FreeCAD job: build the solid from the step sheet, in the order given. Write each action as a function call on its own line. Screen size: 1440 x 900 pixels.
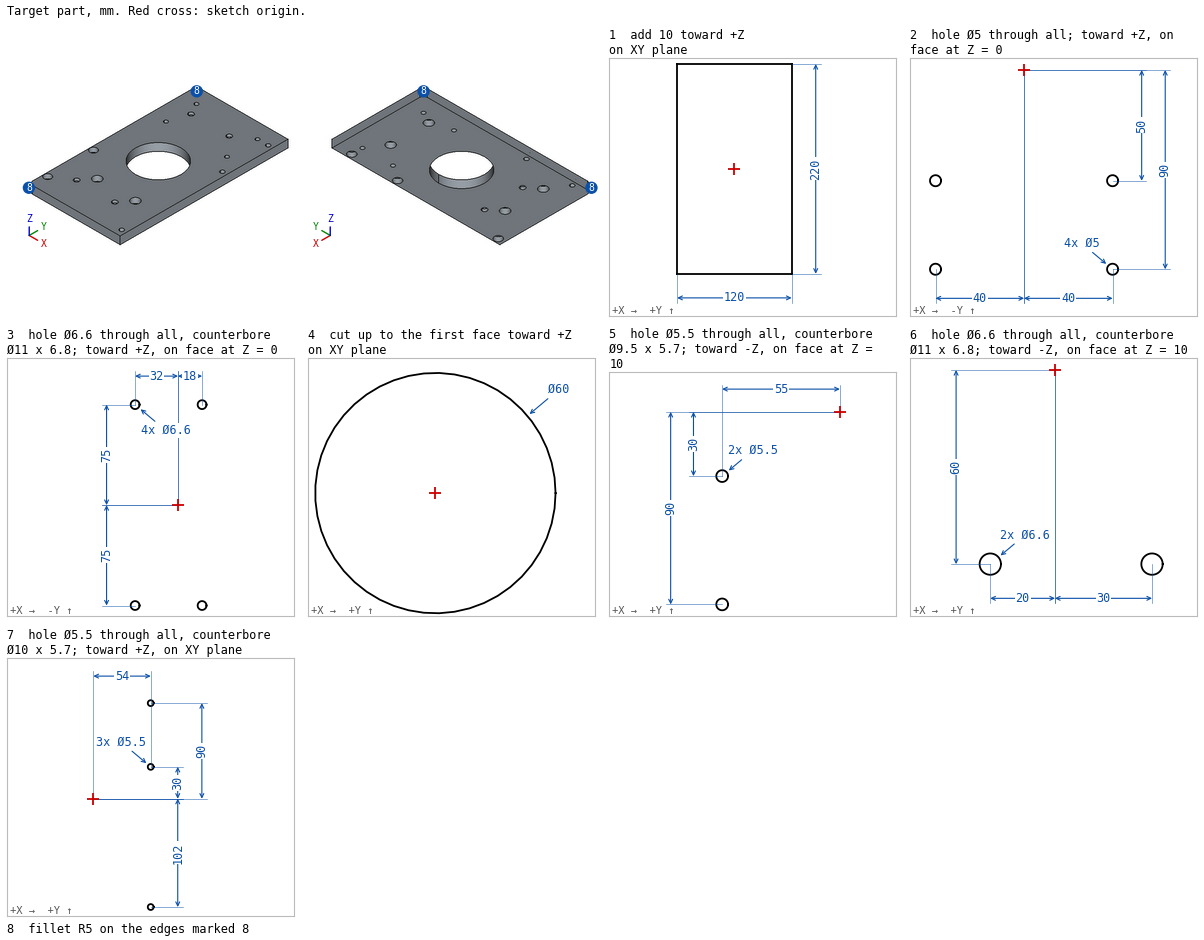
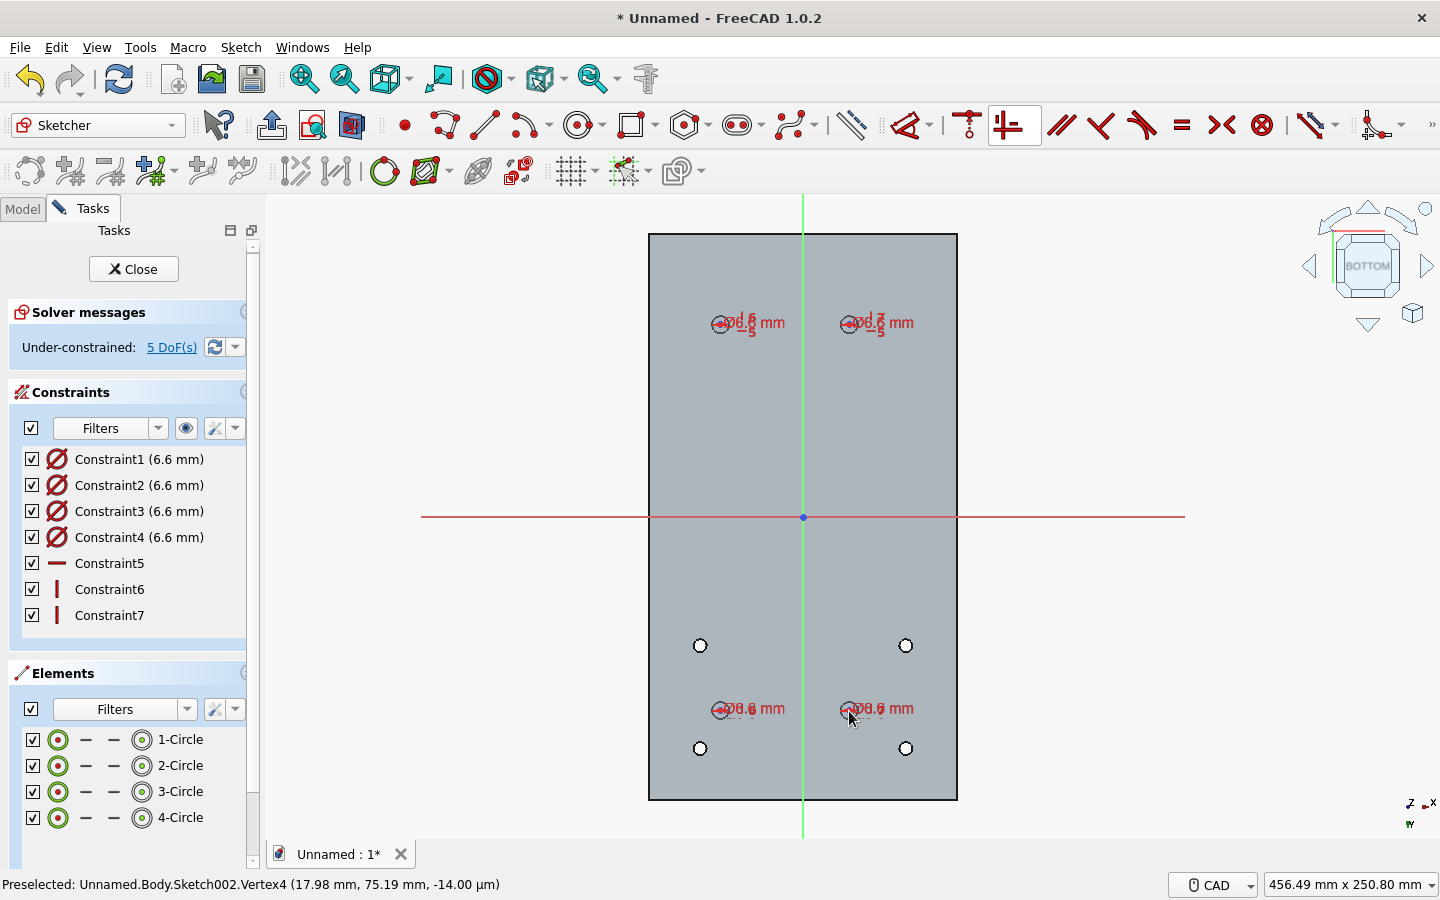
click(721, 711)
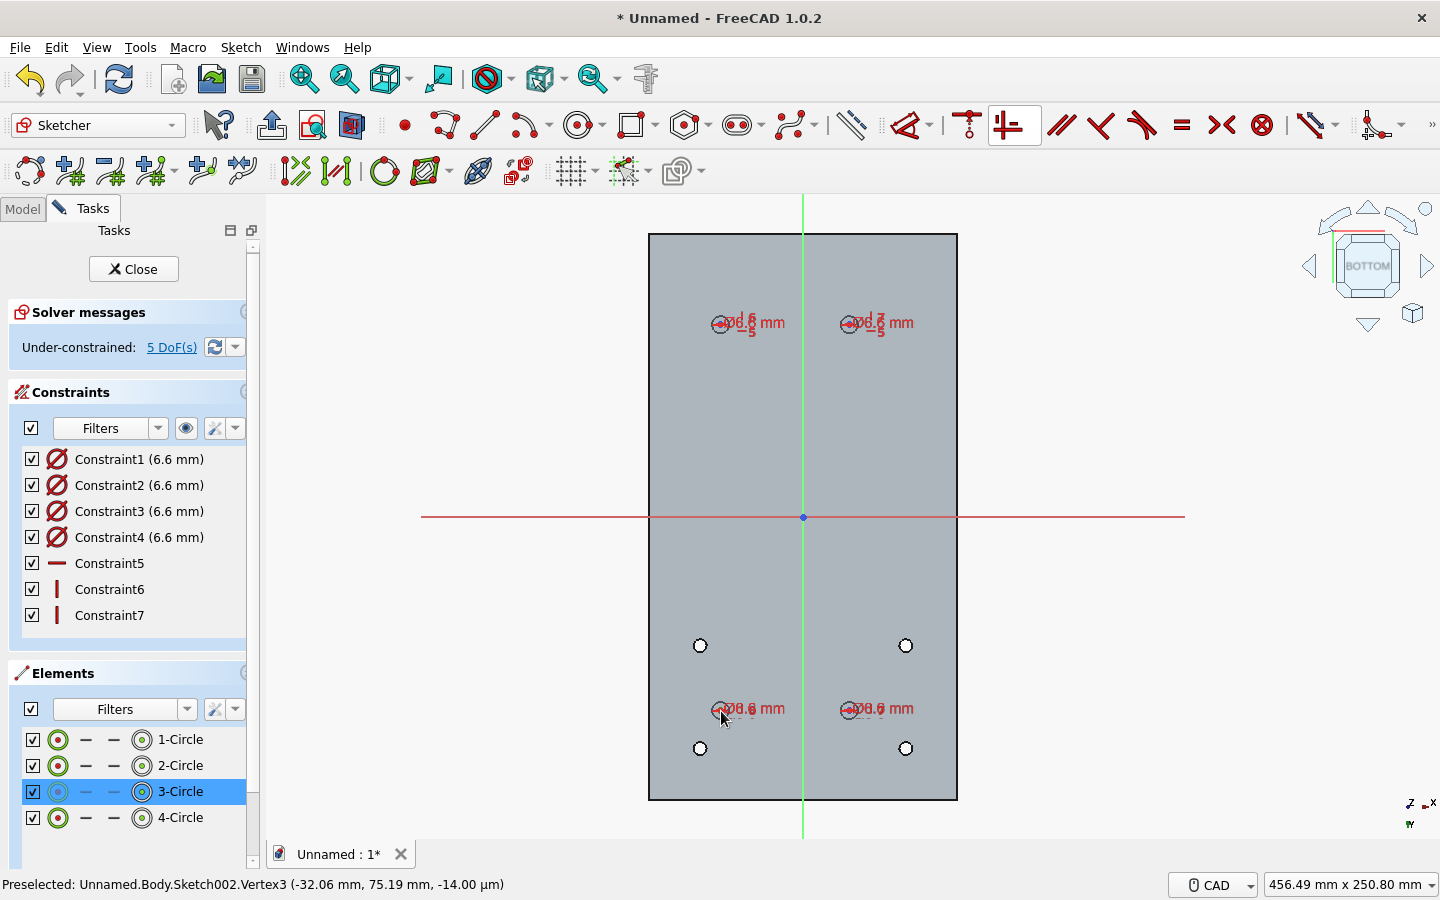
click(849, 711)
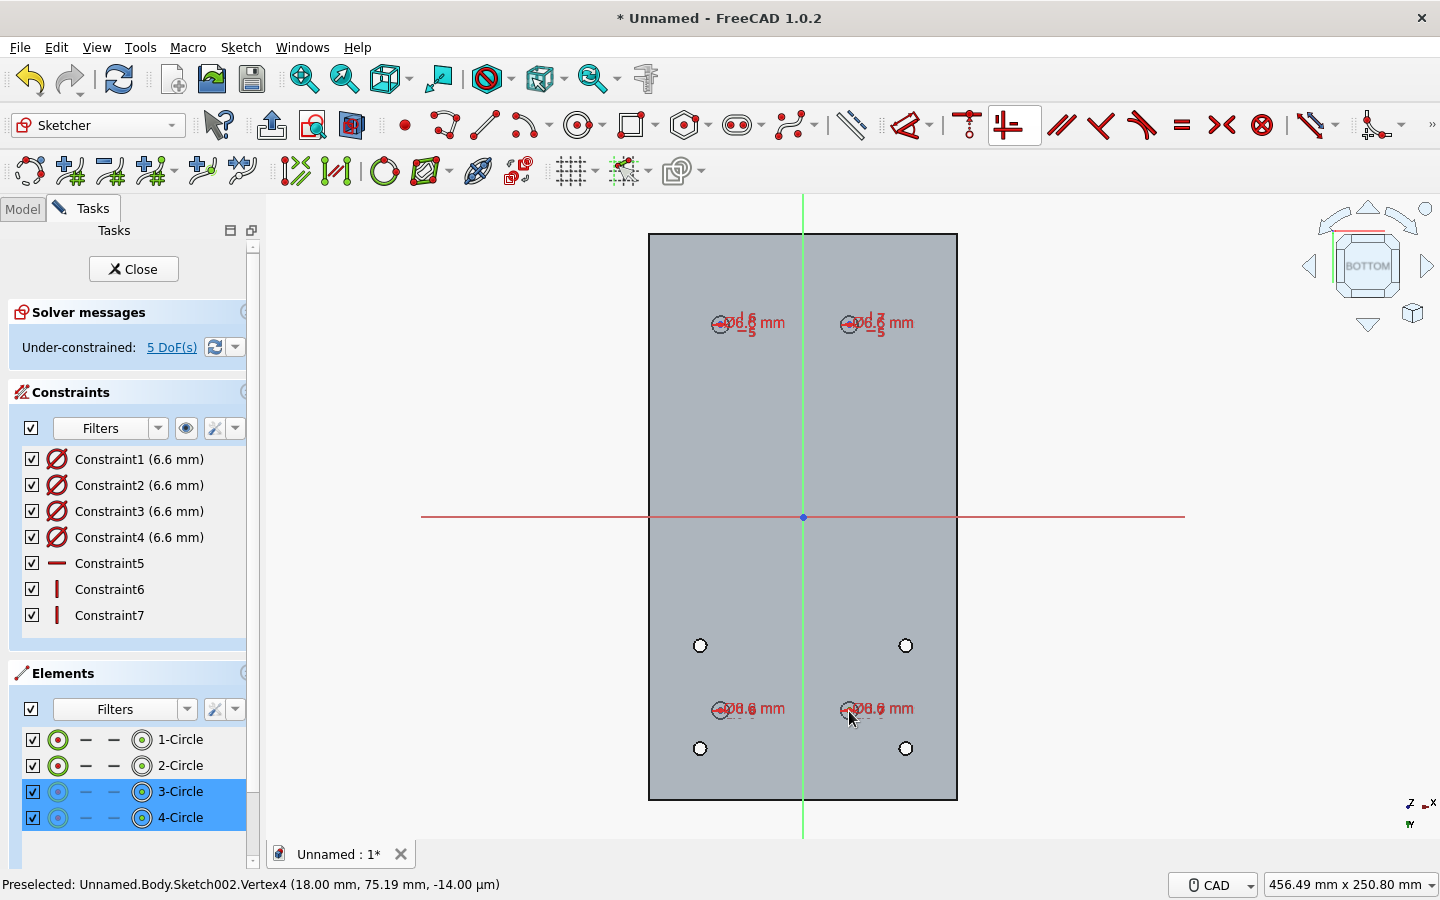
click(1036, 126)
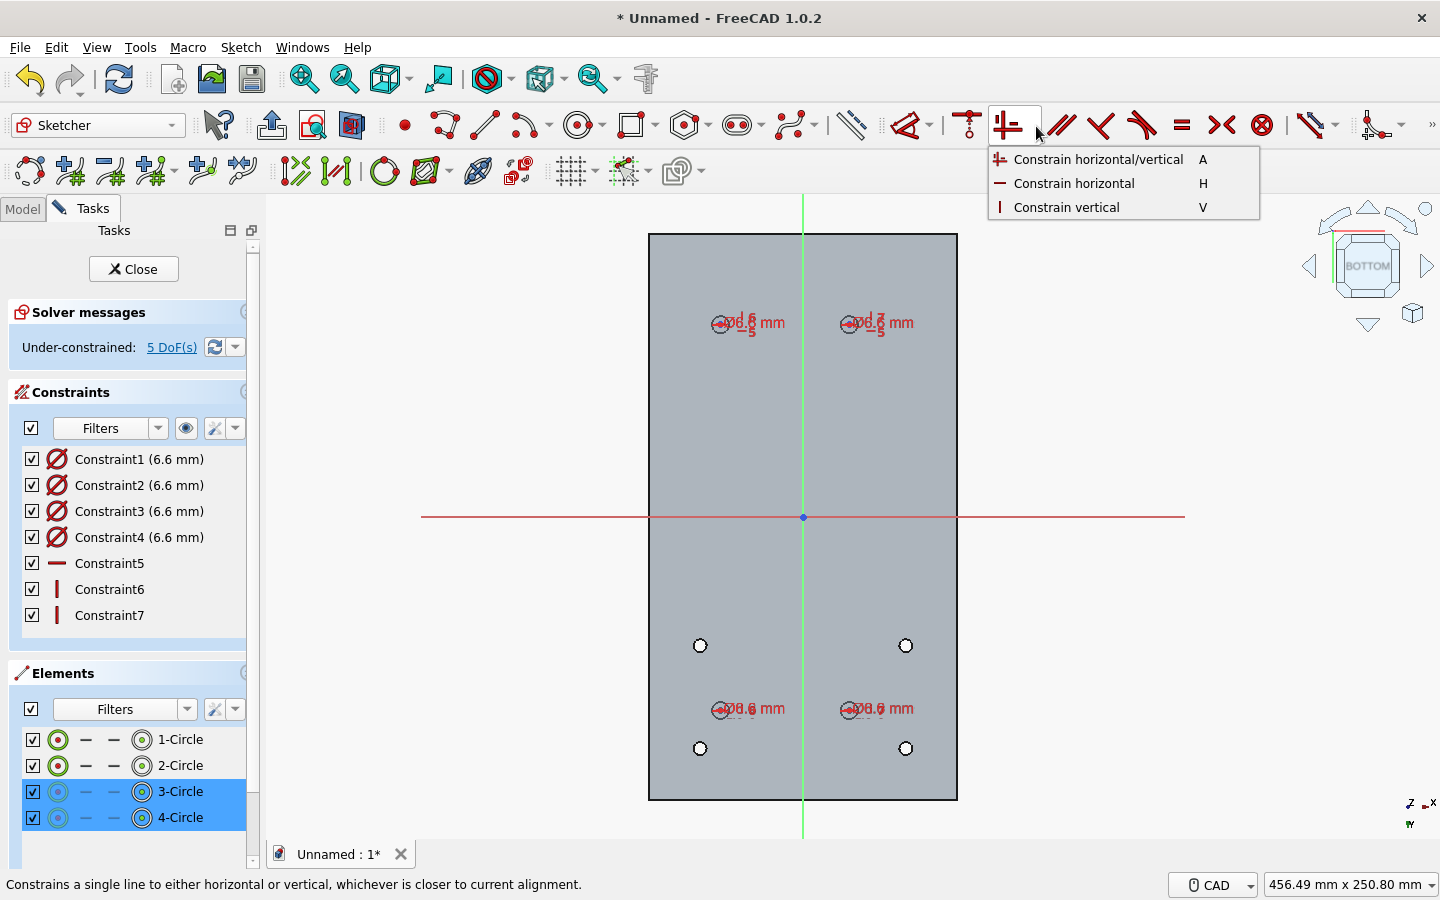
click(1124, 183)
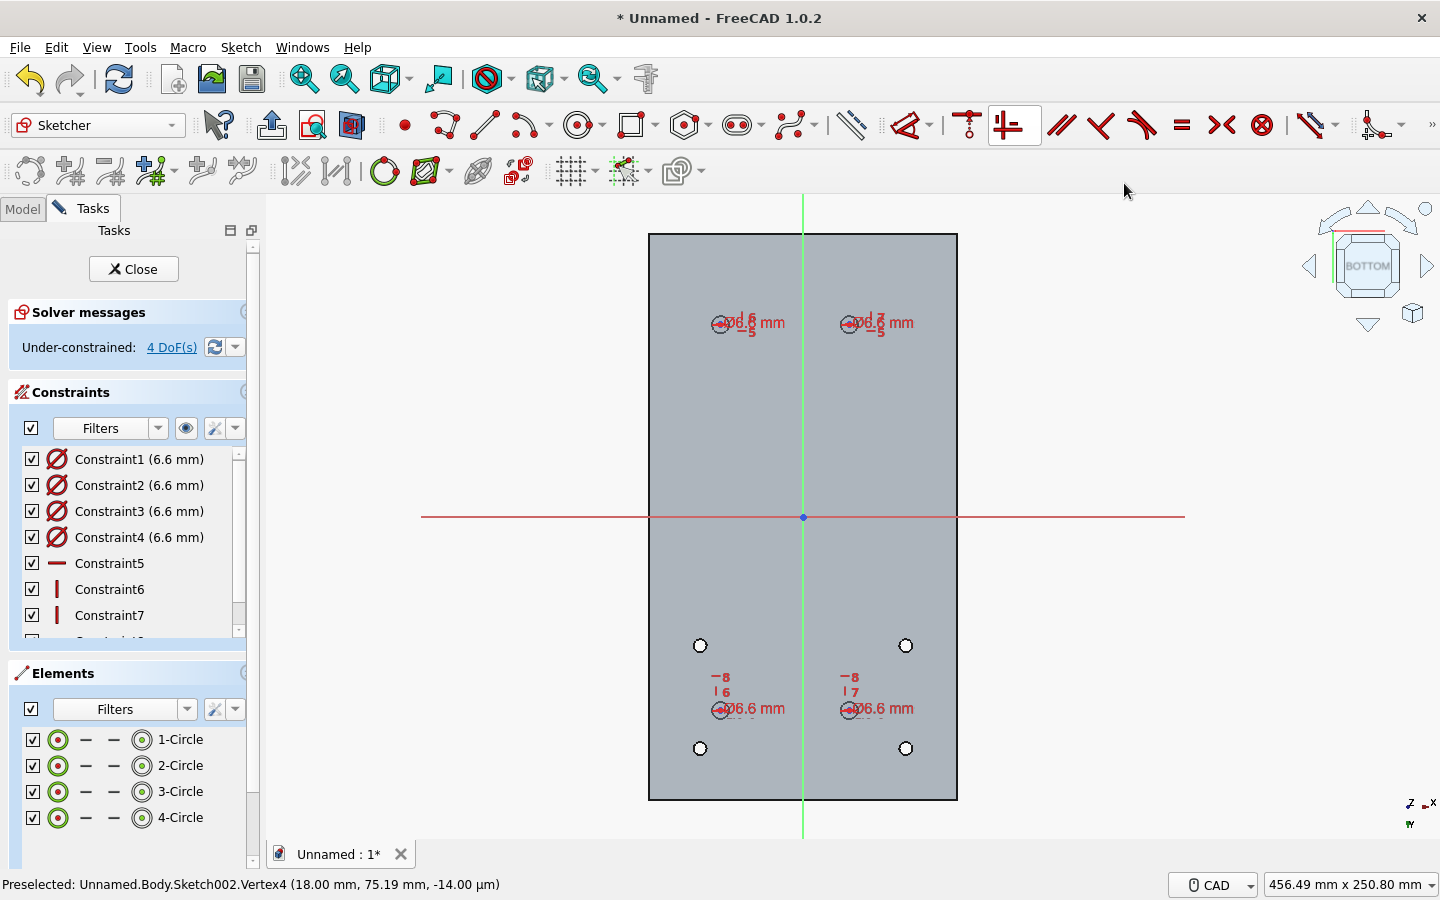
click(906, 126)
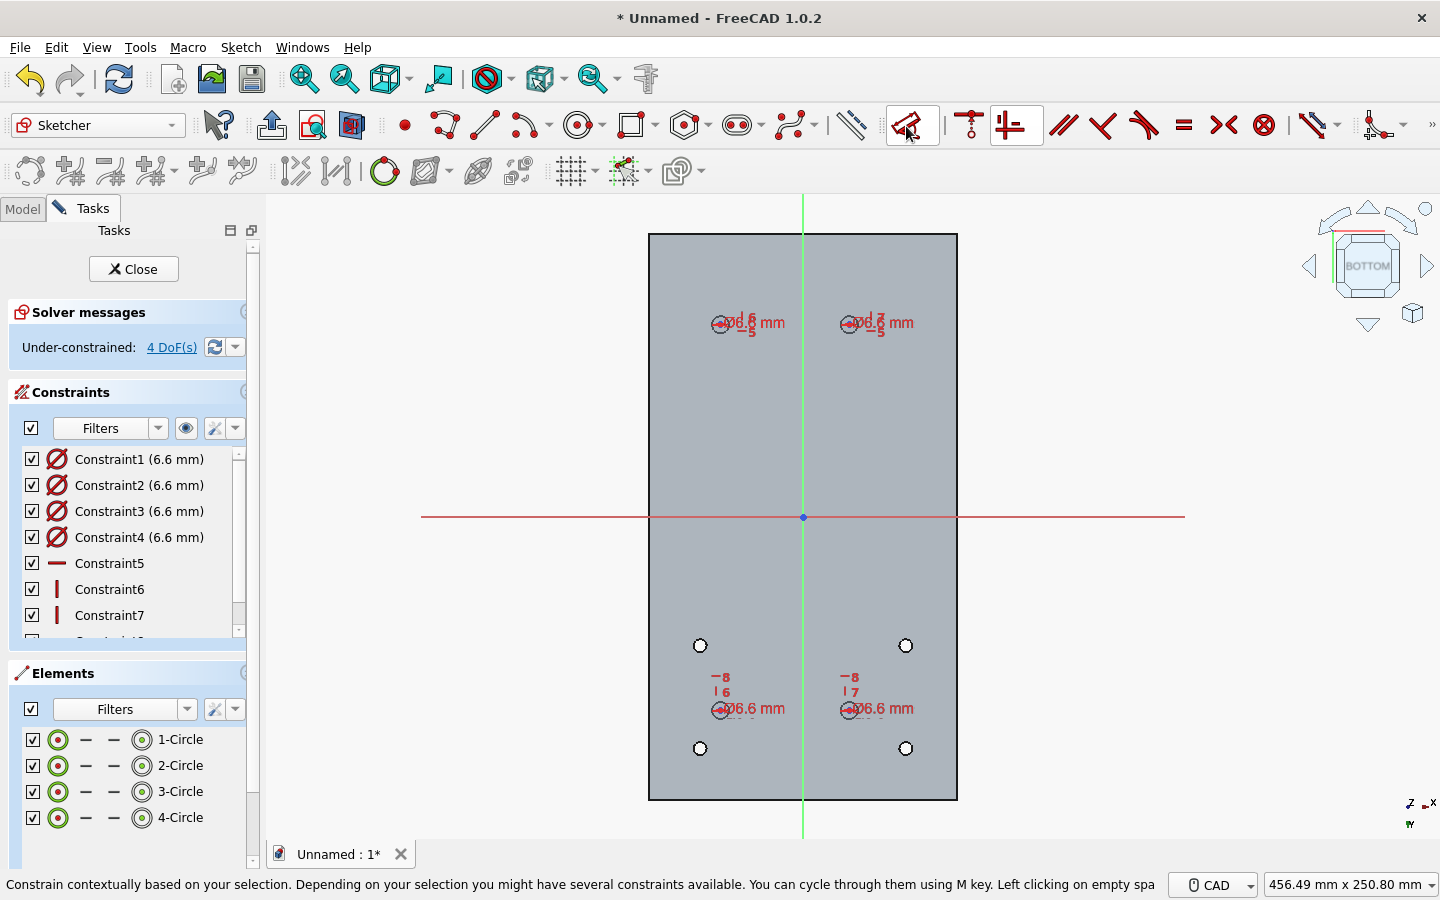
click(721, 325)
click(762, 291)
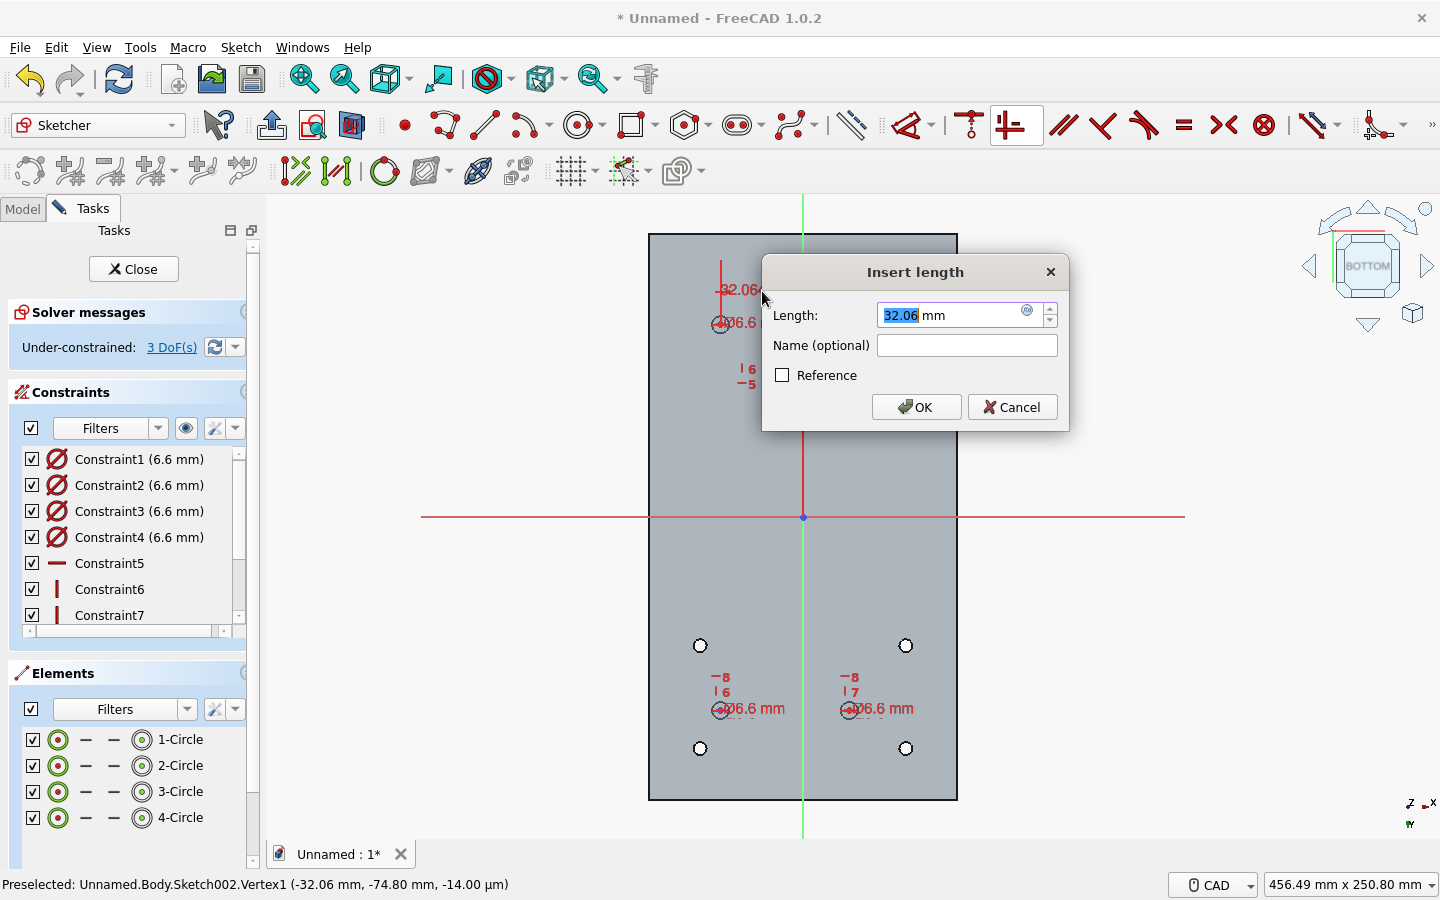
text(32)
key(Return)